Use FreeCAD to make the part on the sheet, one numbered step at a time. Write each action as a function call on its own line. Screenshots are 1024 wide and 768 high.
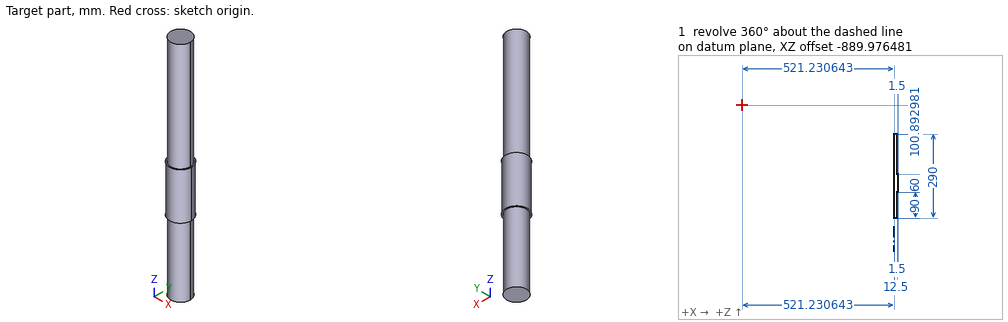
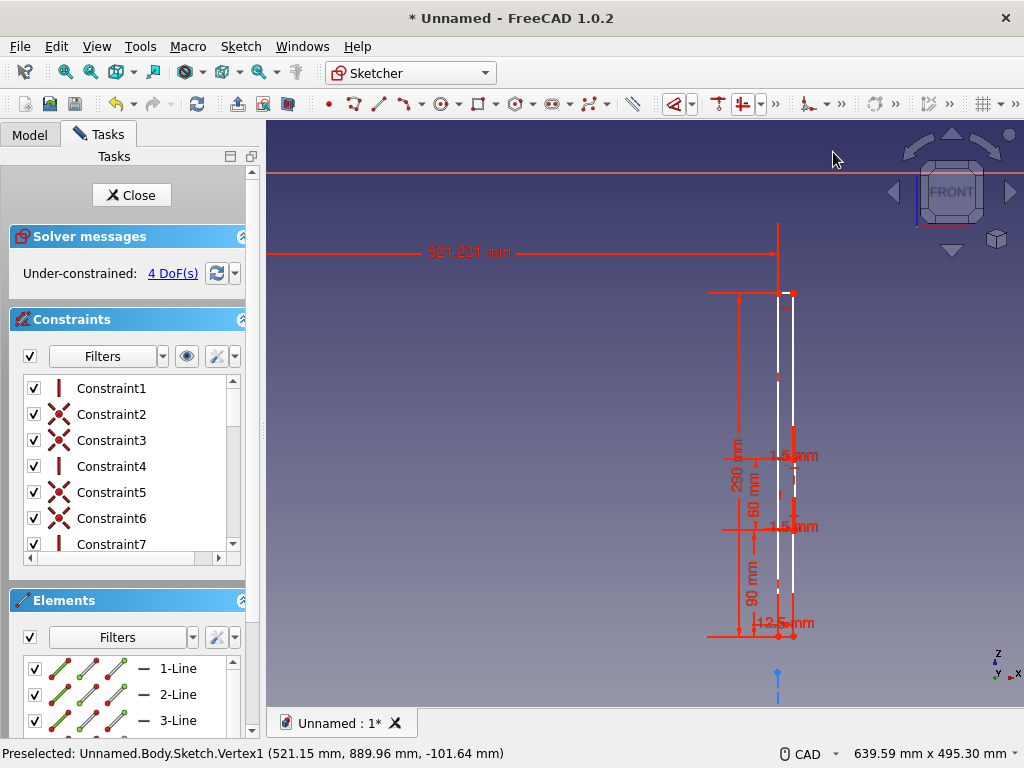
click(778, 293)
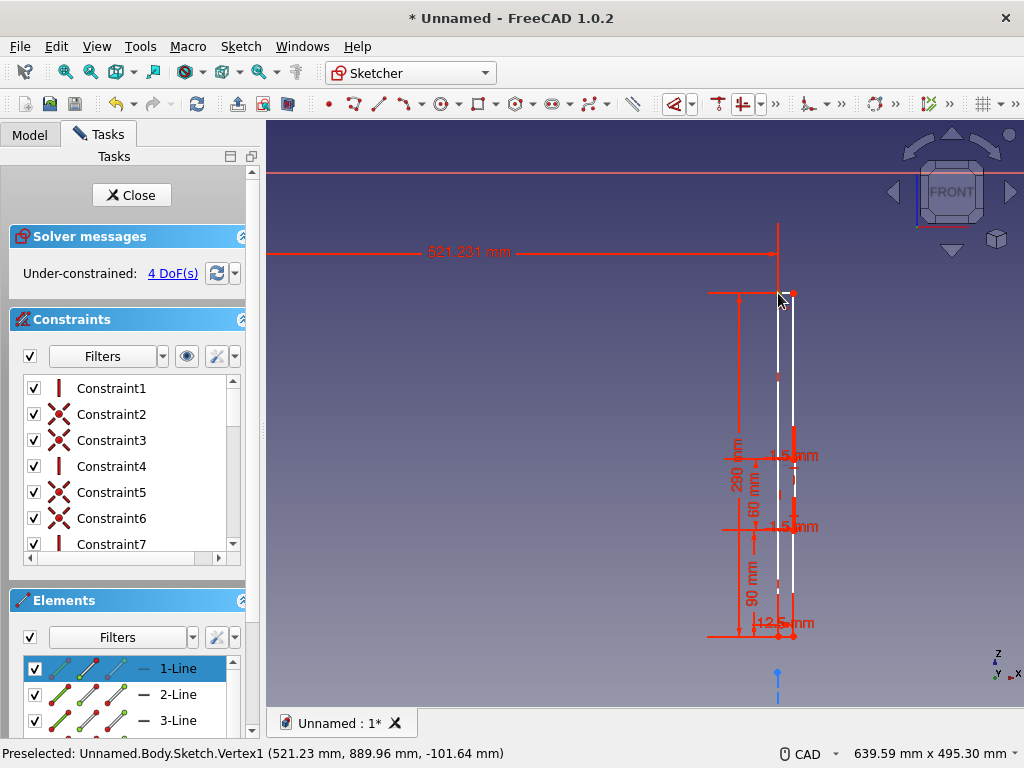
key(i)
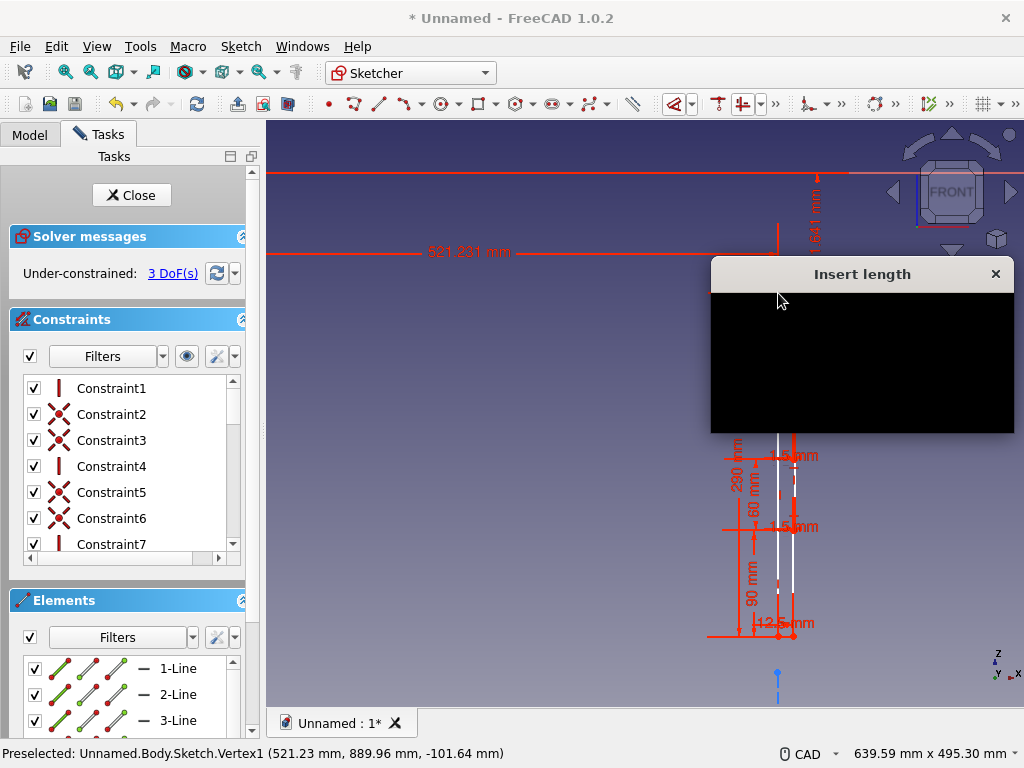
text(-100.892981)
key(Return)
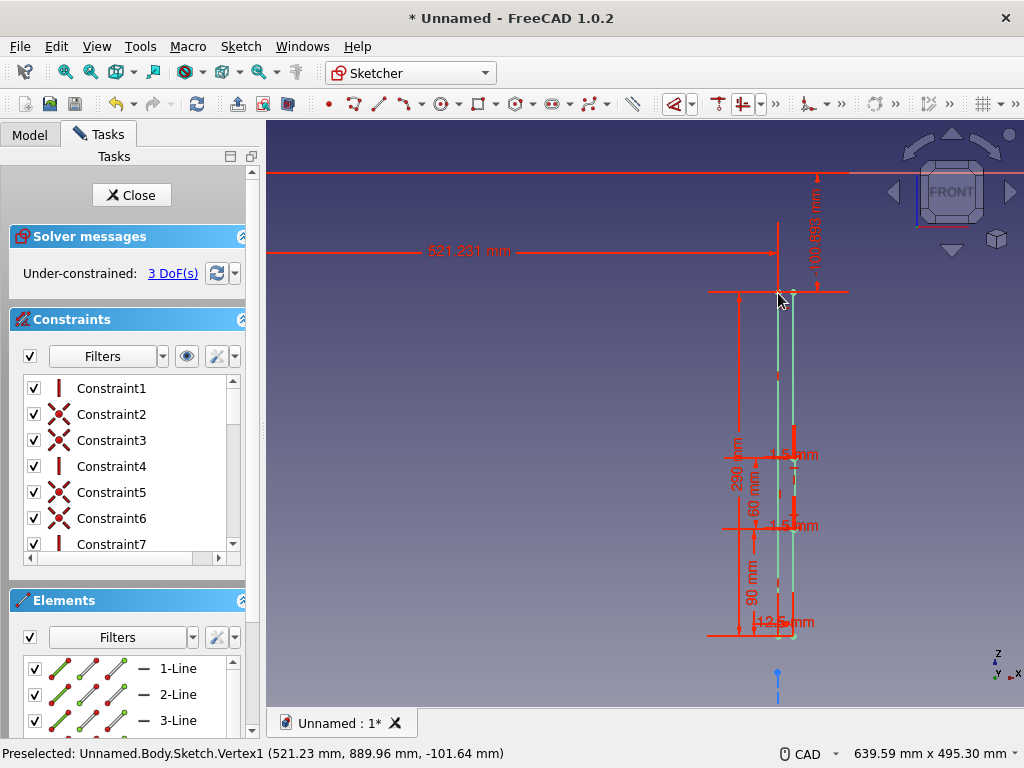
click(778, 672)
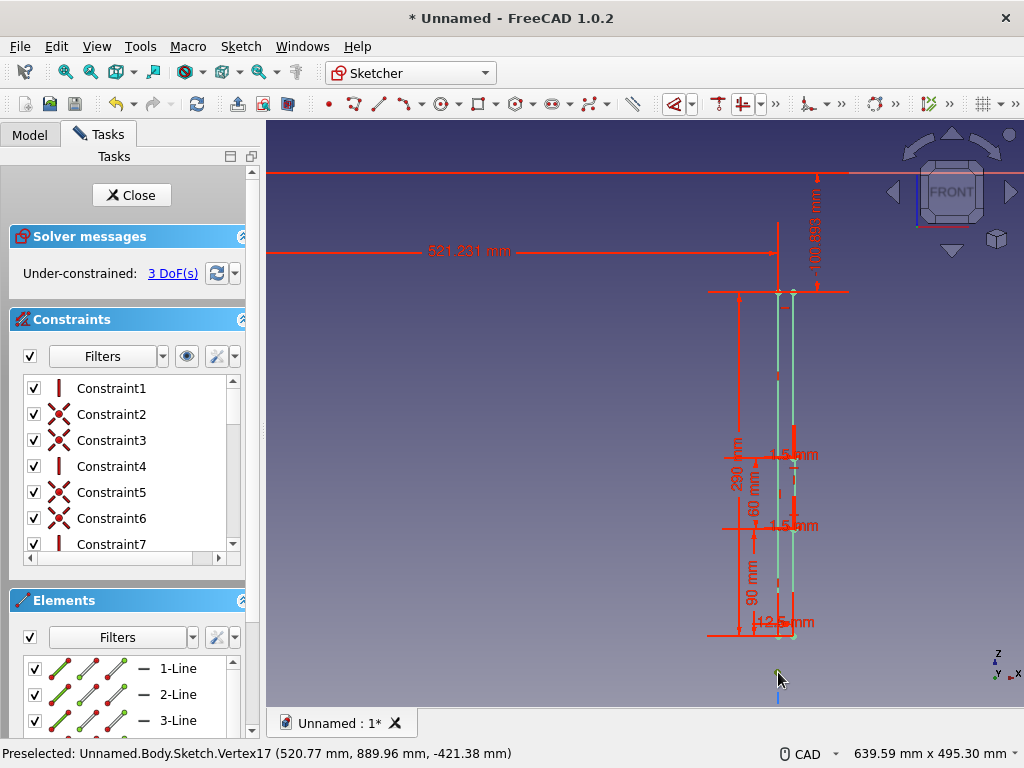
key(l)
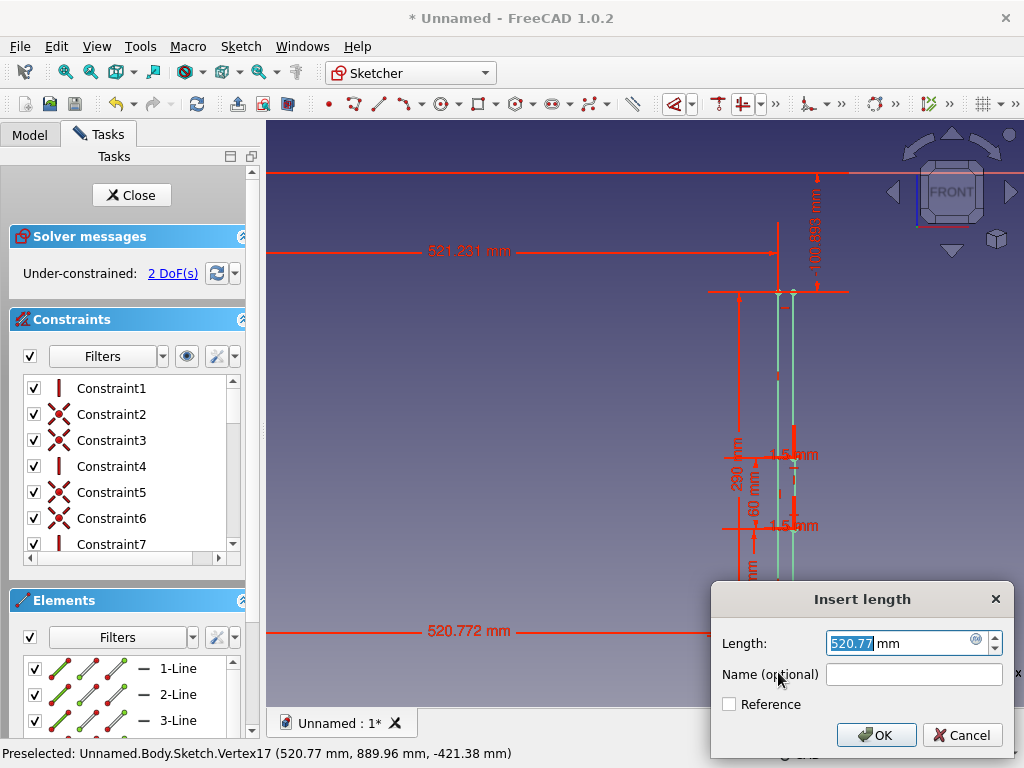
text(521.230643)
key(Return)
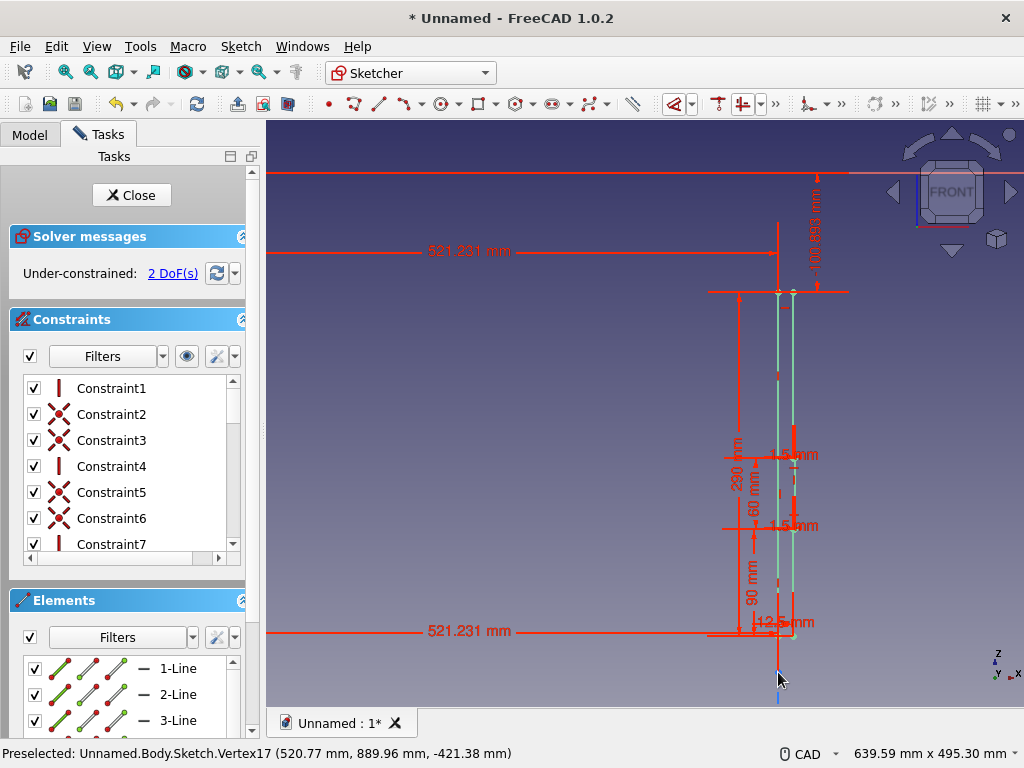
click(132, 195)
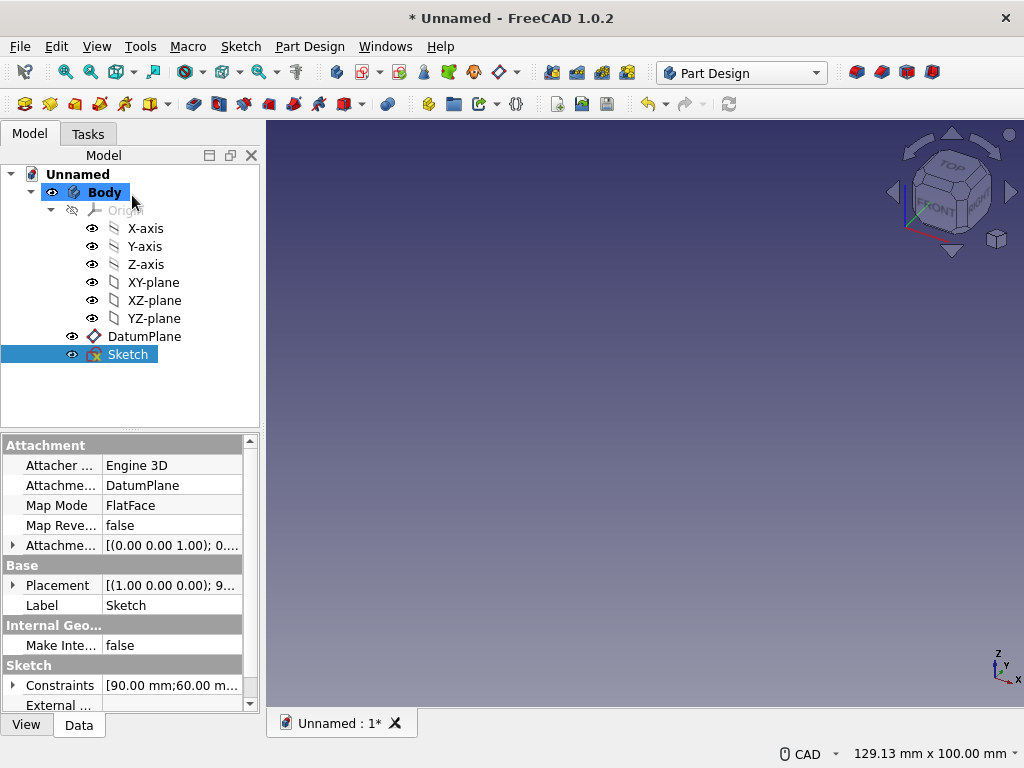
click(50, 104)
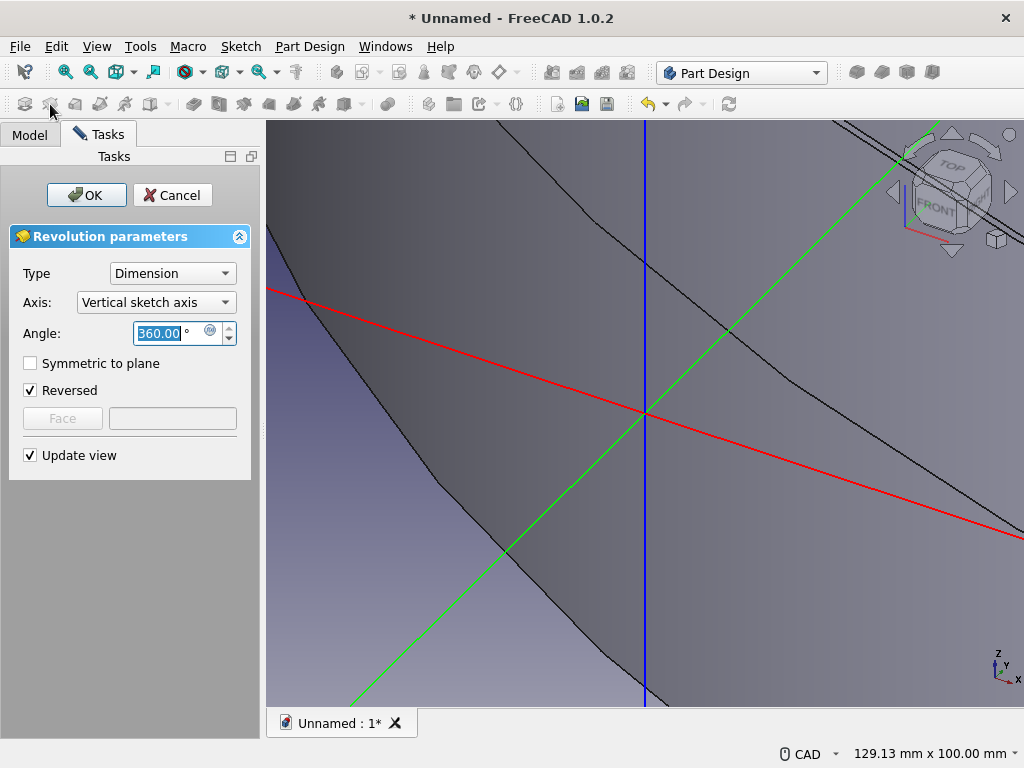
click(157, 302)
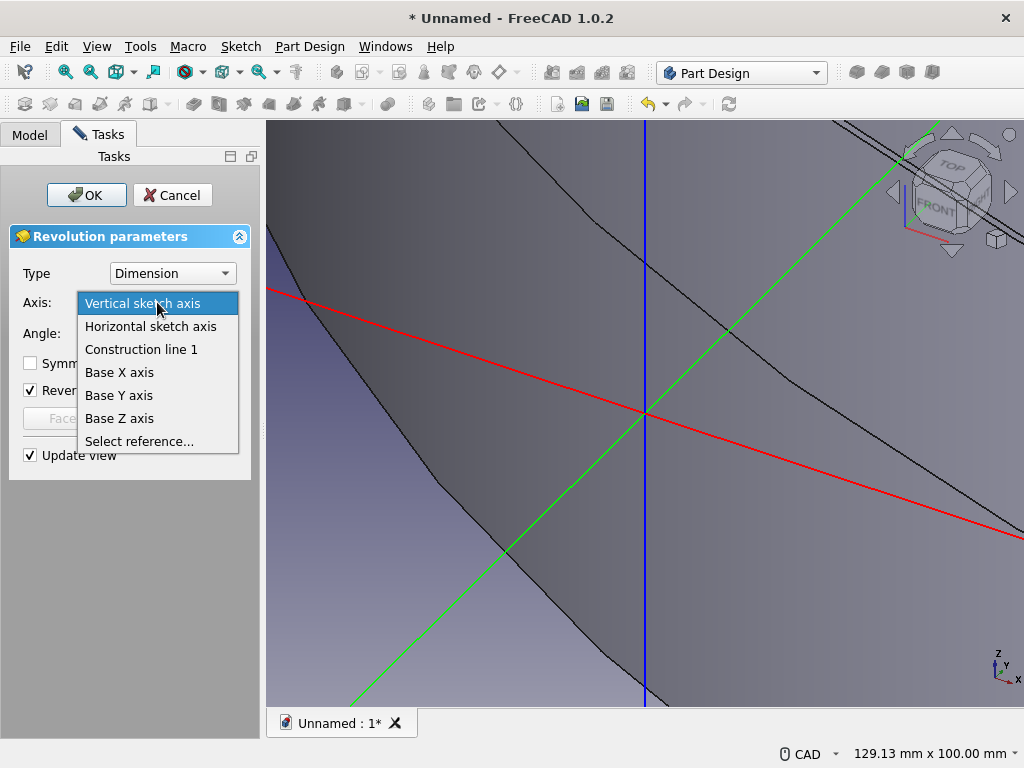
click(156, 350)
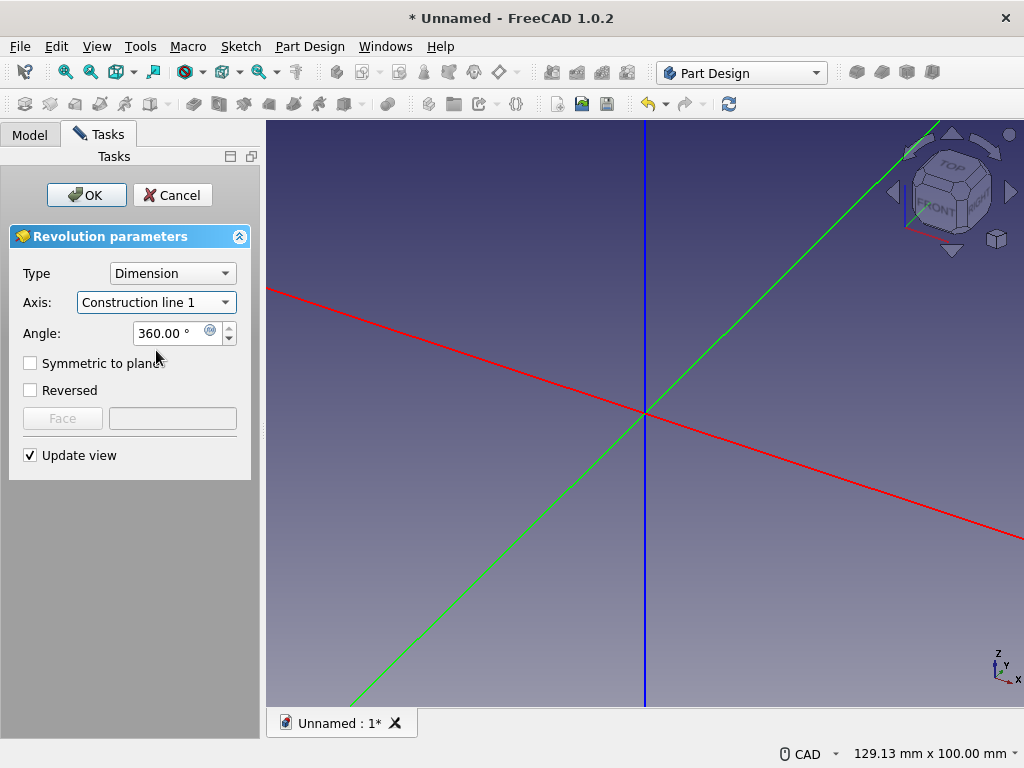
click(87, 195)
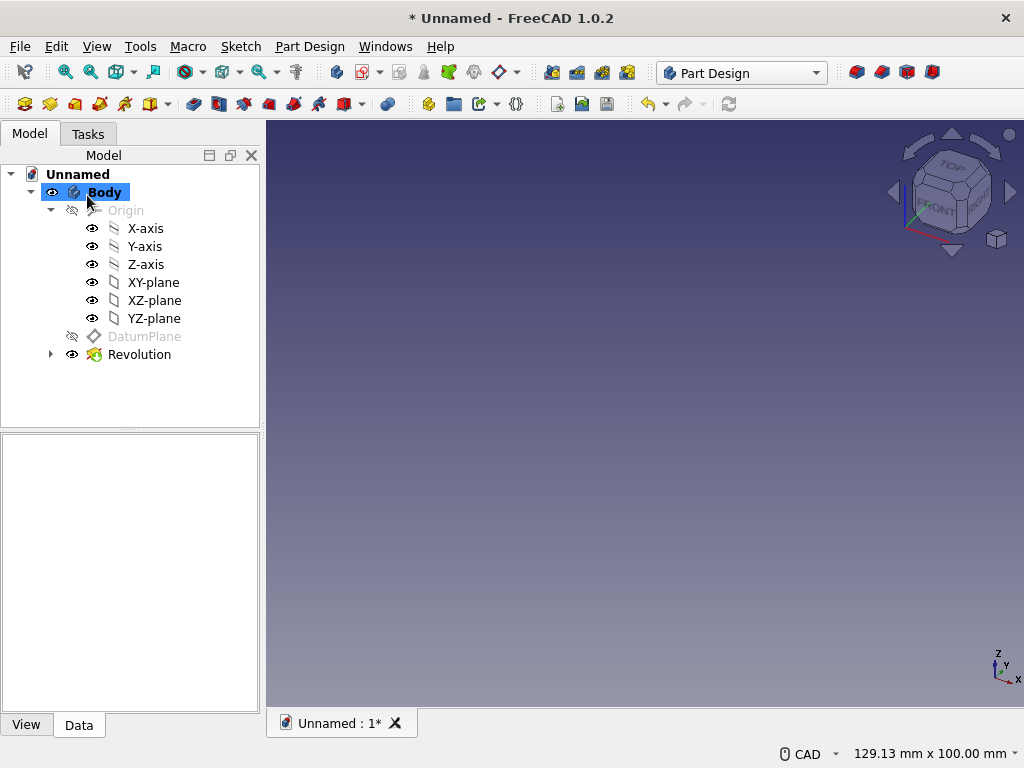
key(0)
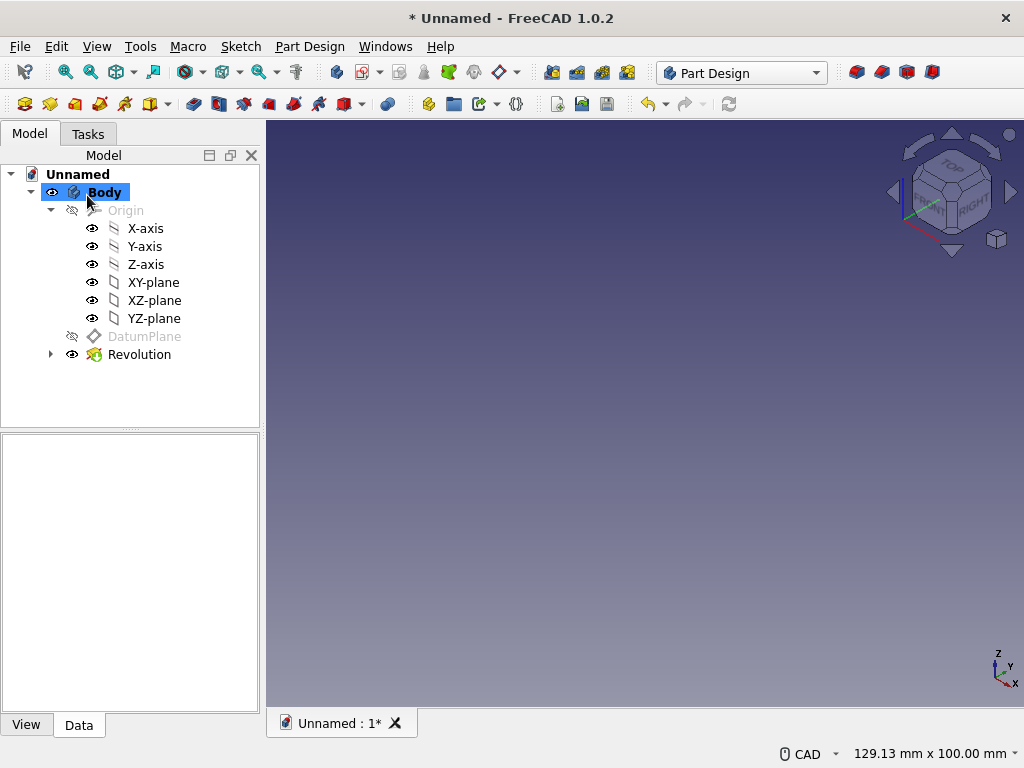
click(66, 72)